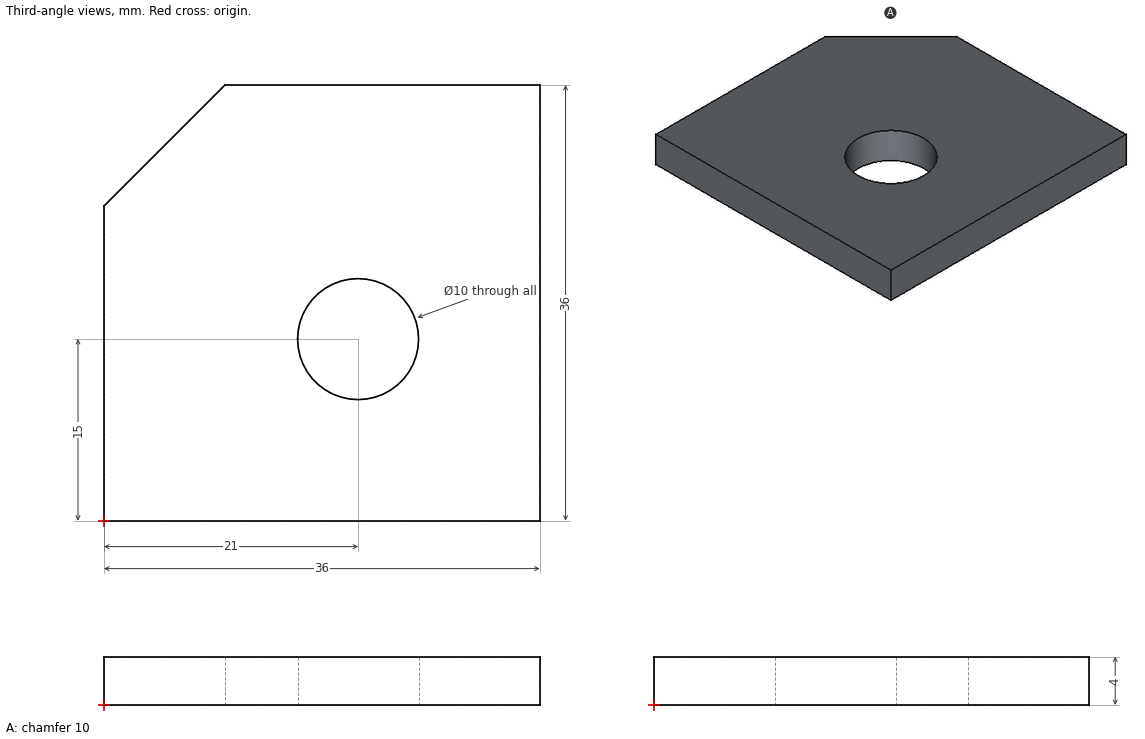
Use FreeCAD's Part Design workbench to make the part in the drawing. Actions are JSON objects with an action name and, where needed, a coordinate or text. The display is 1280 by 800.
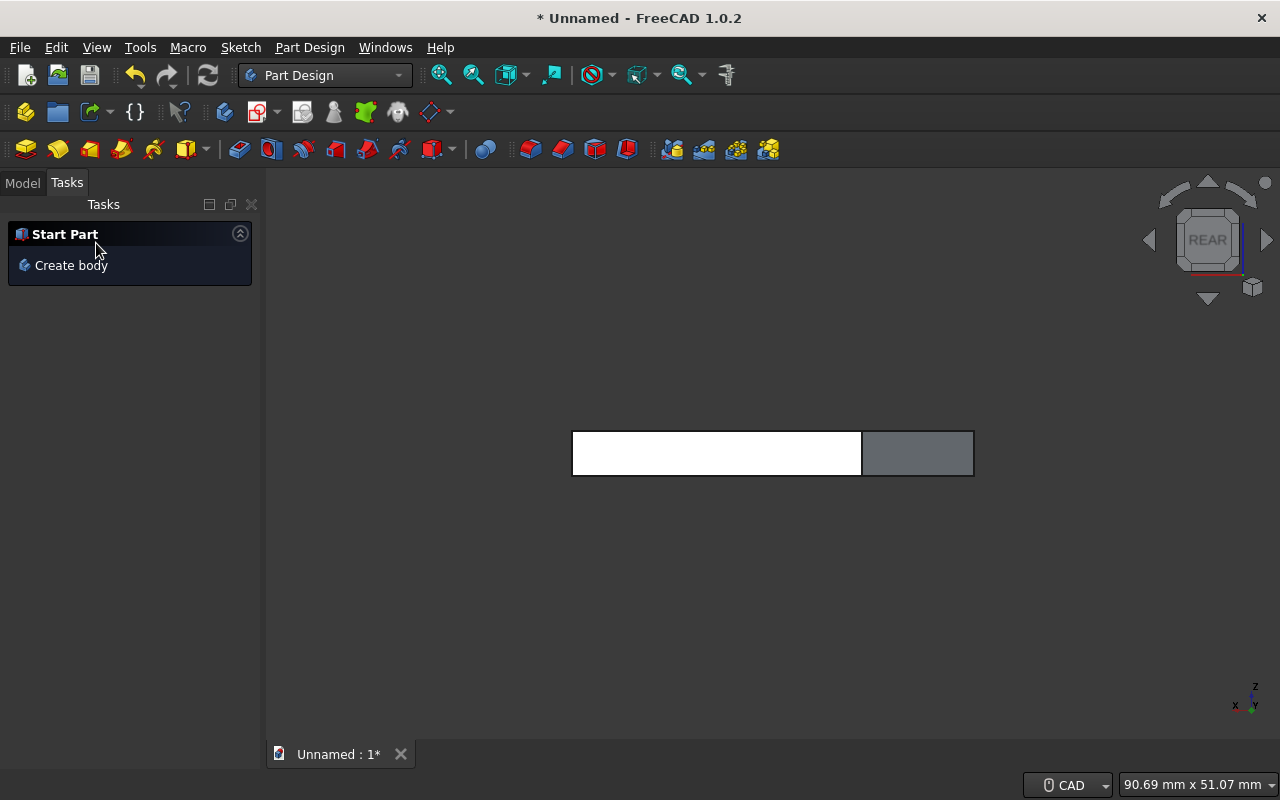
{"action": "key", "text": "v f"}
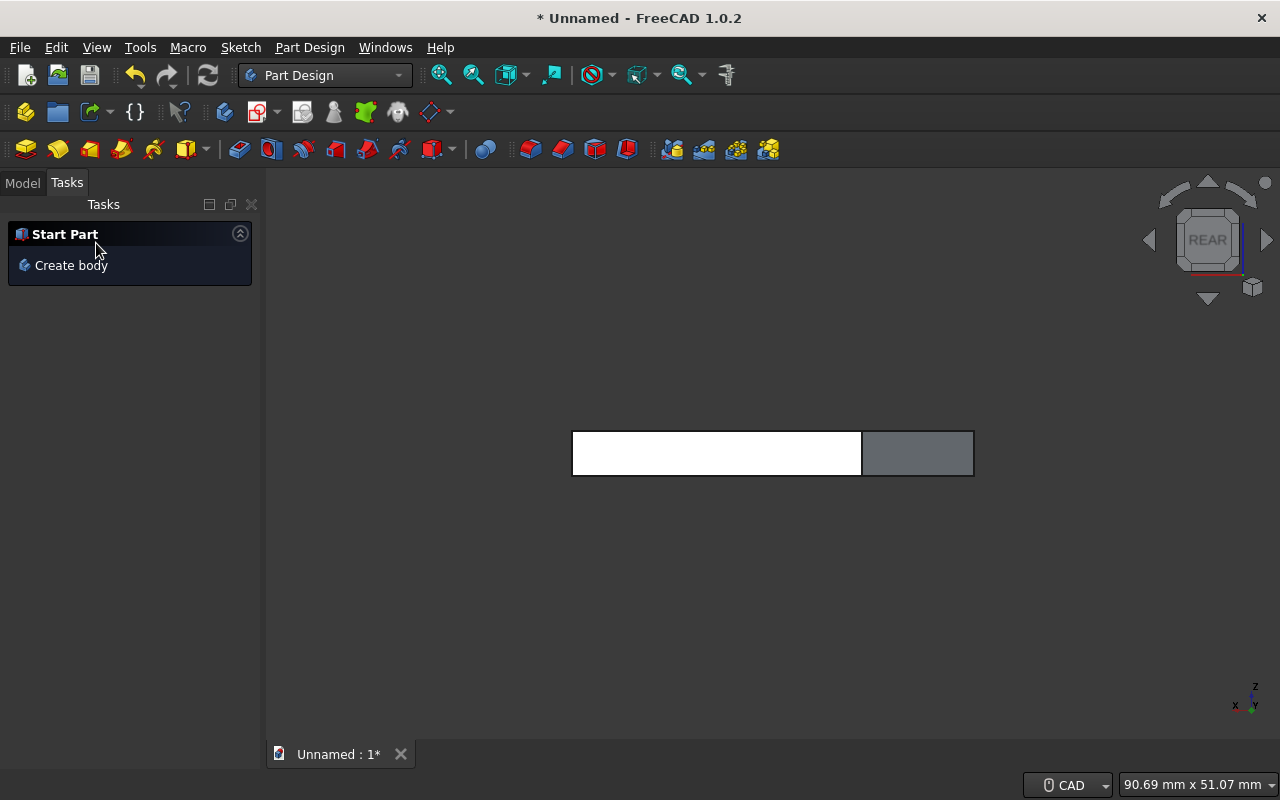
{"action": "key", "text": "0"}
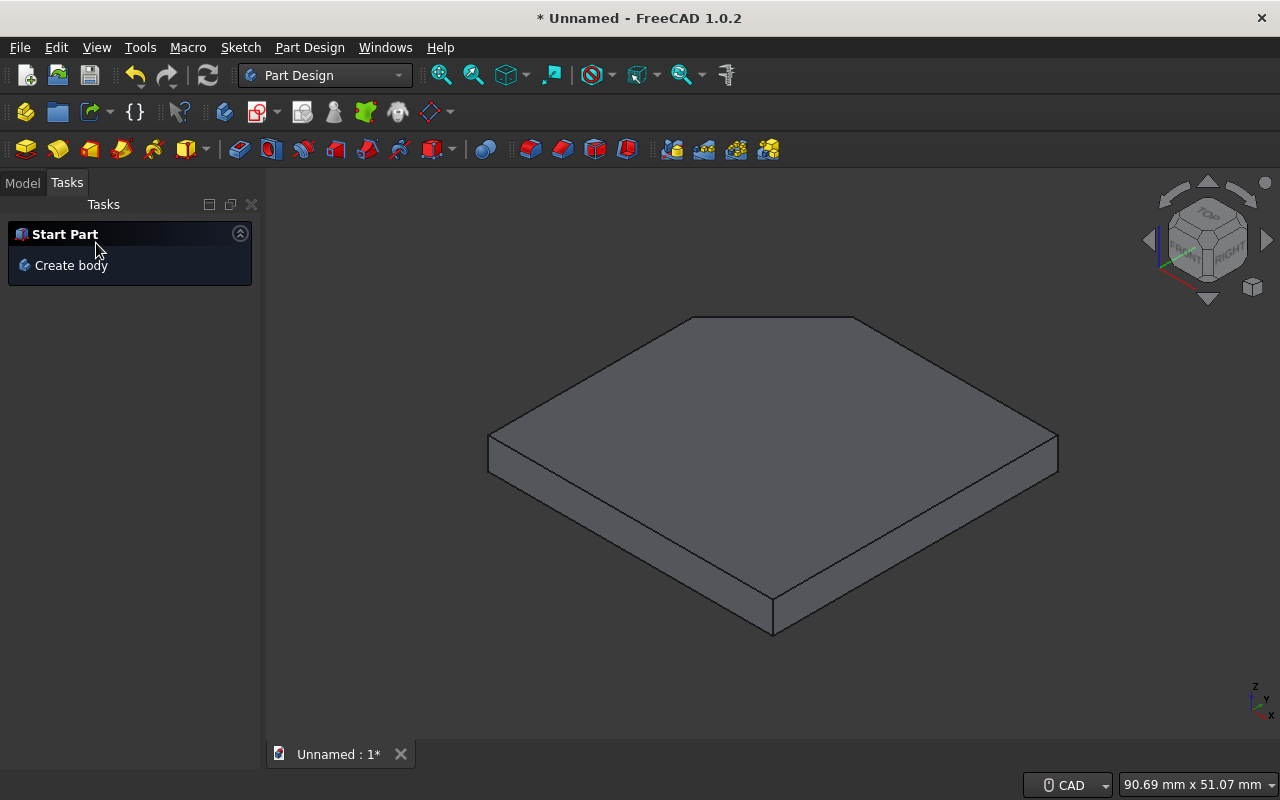
{"action": "left_click", "coordinate": [773, 434]}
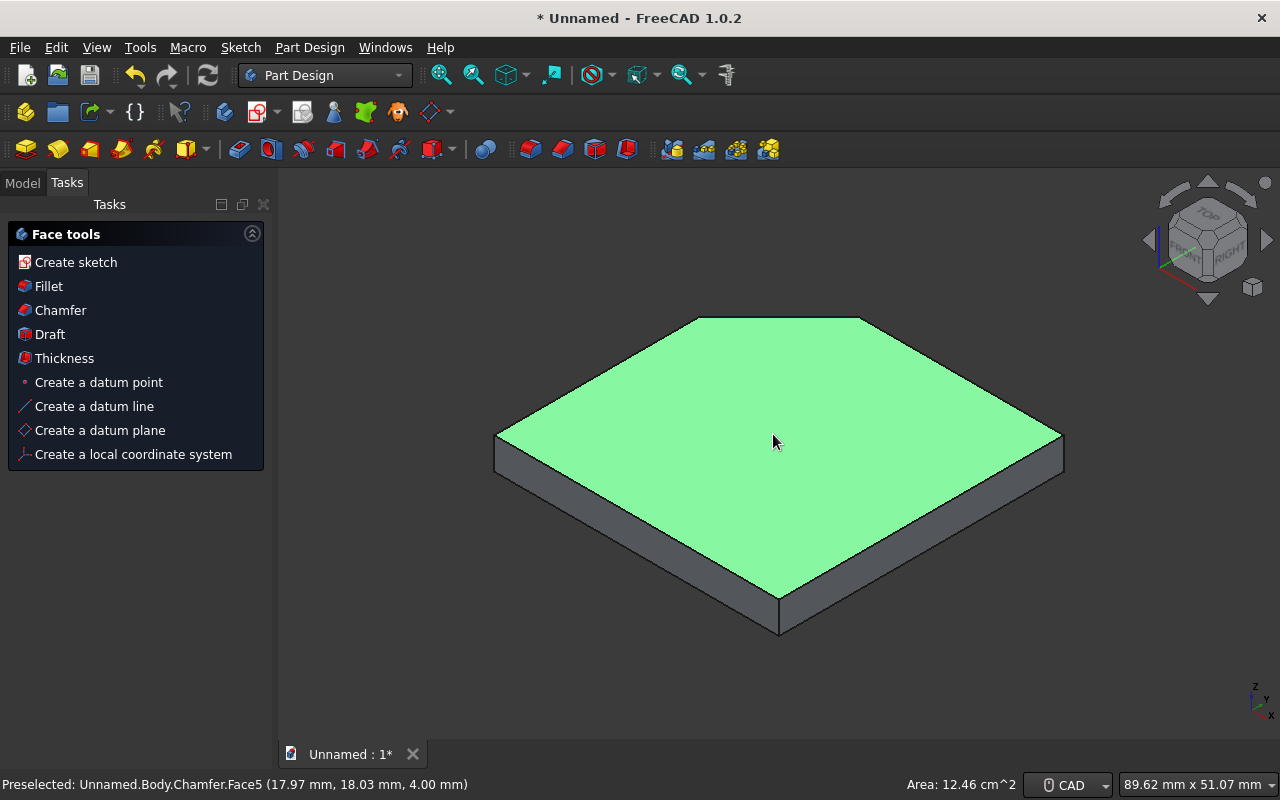
{"action": "left_click", "coordinate": [258, 112]}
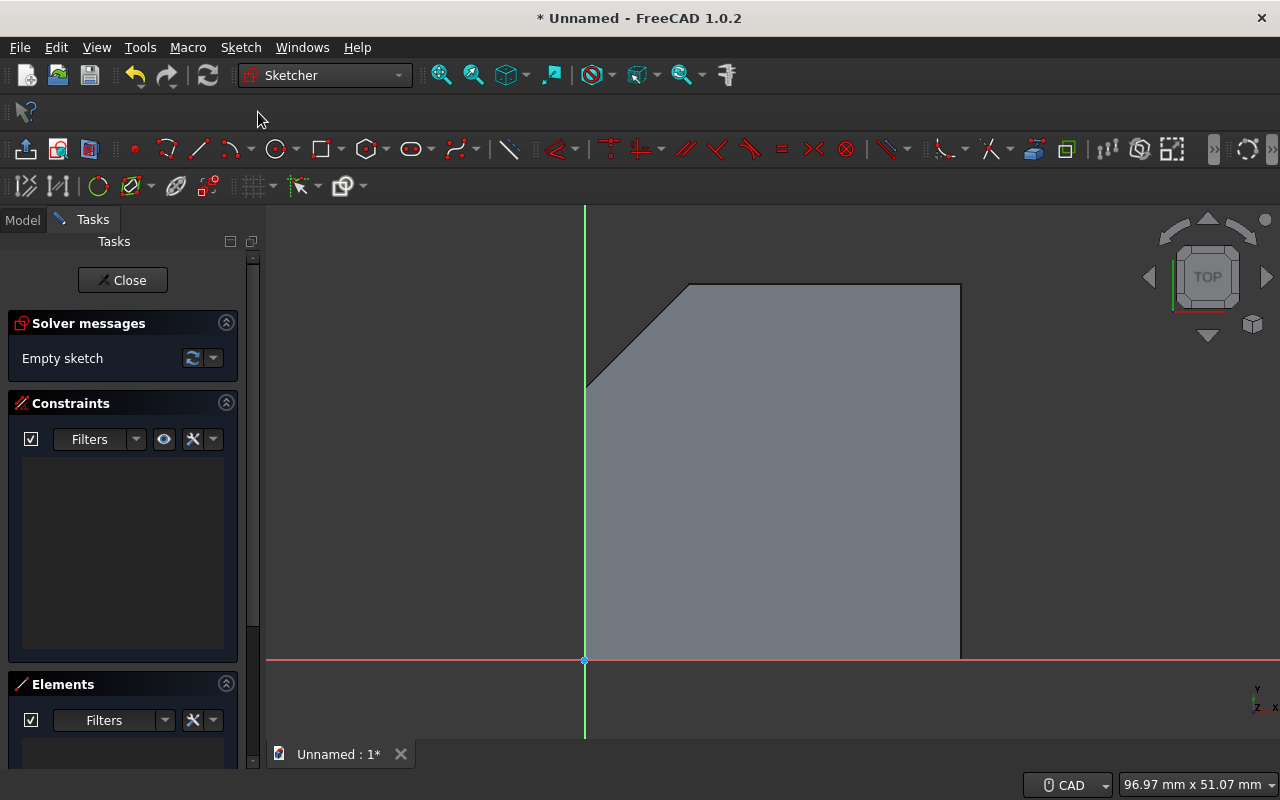
{"action": "scroll", "coordinate": [847, 517], "scroll_direction": "up", "scroll_amount": 6}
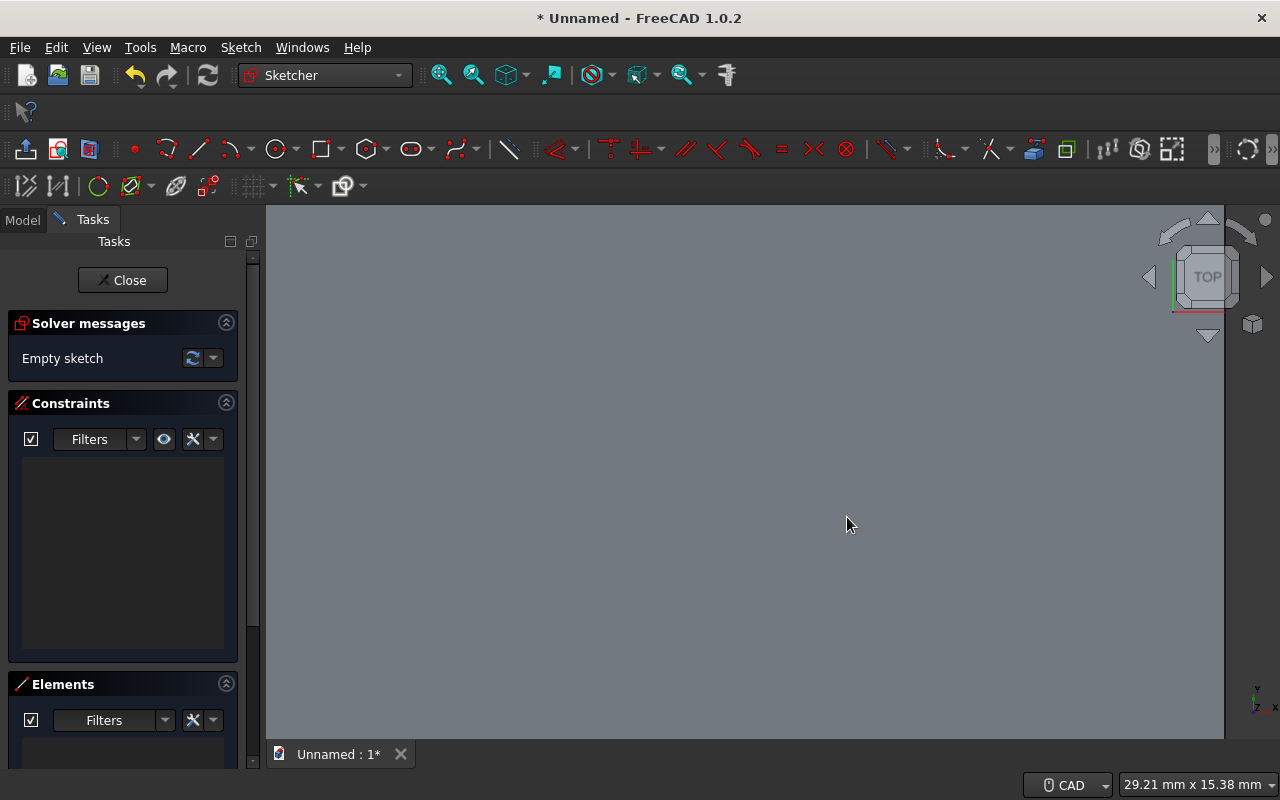
{"action": "key", "text": "g c"}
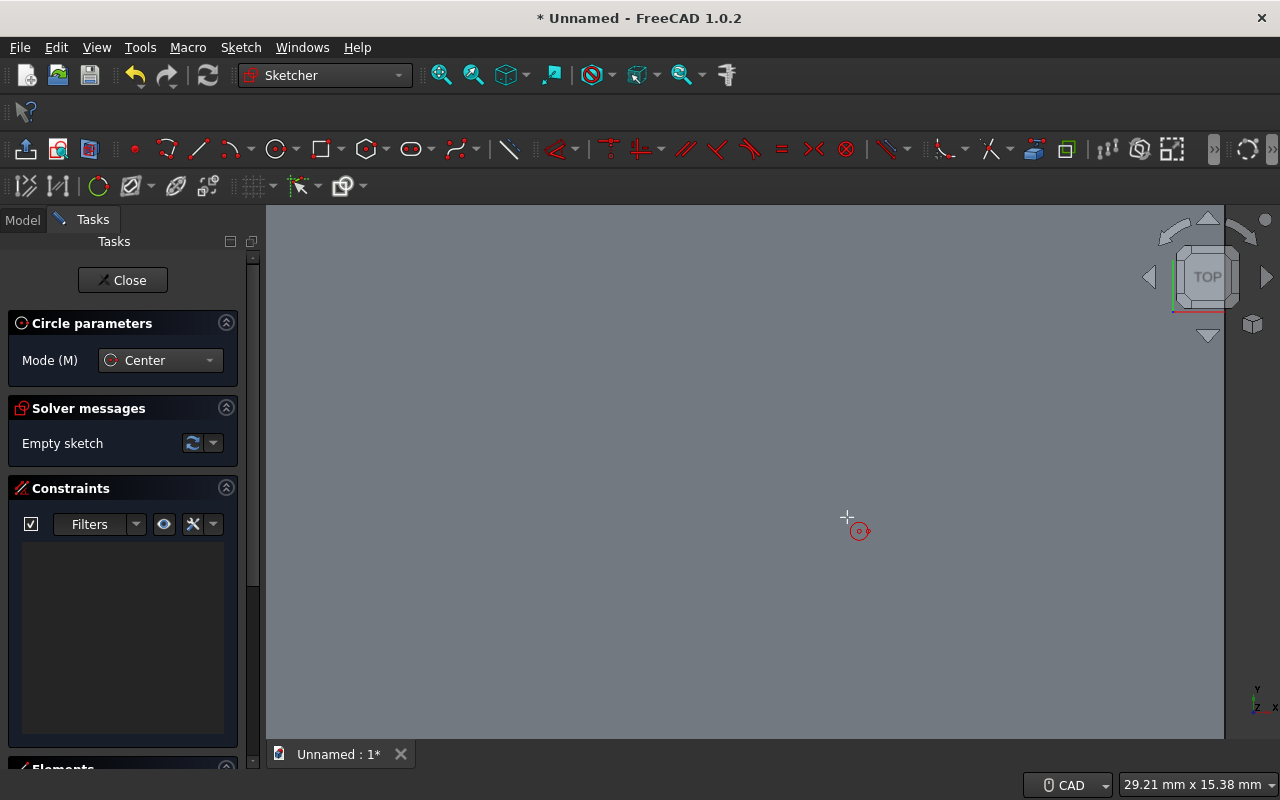
{"action": "left_click", "coordinate": [704, 470]}
{"action": "left_click", "coordinate": [827, 348]}
{"action": "key", "text": "Escape"}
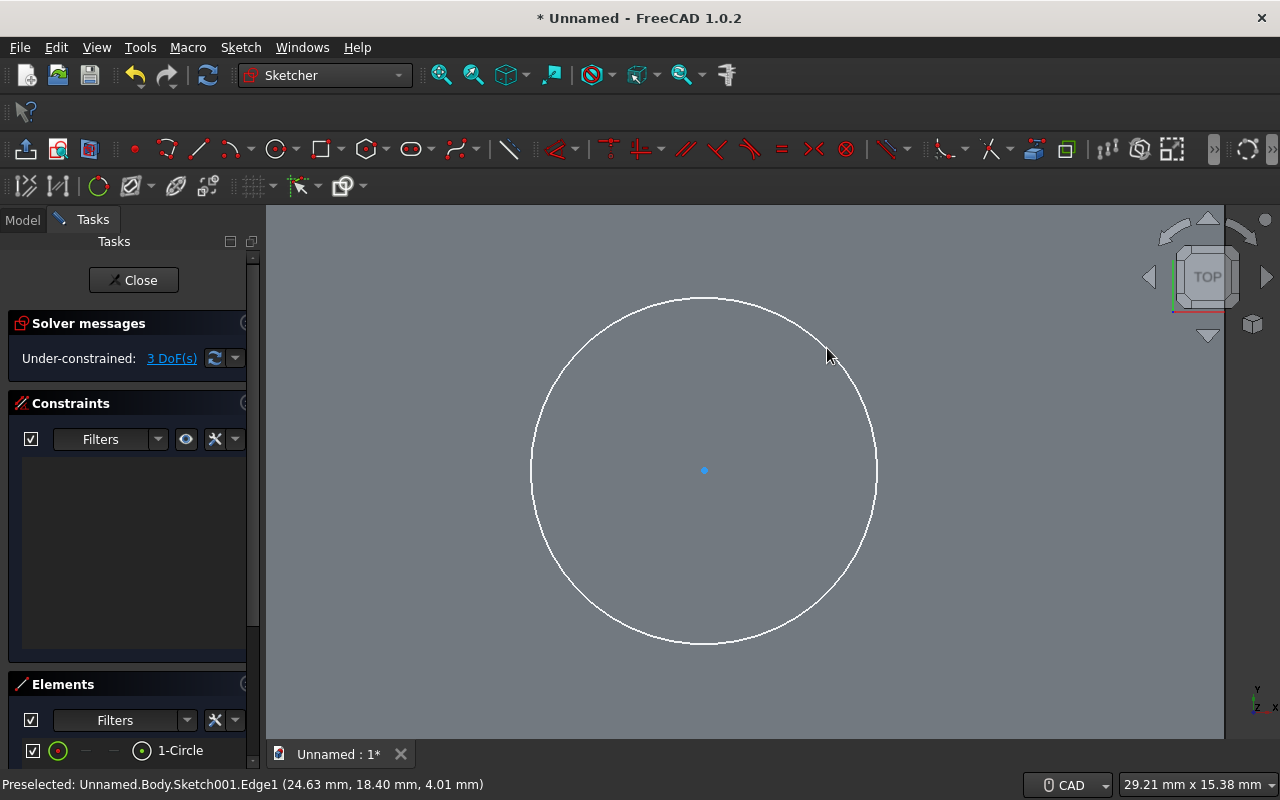
{"action": "left_click", "coordinate": [556, 150]}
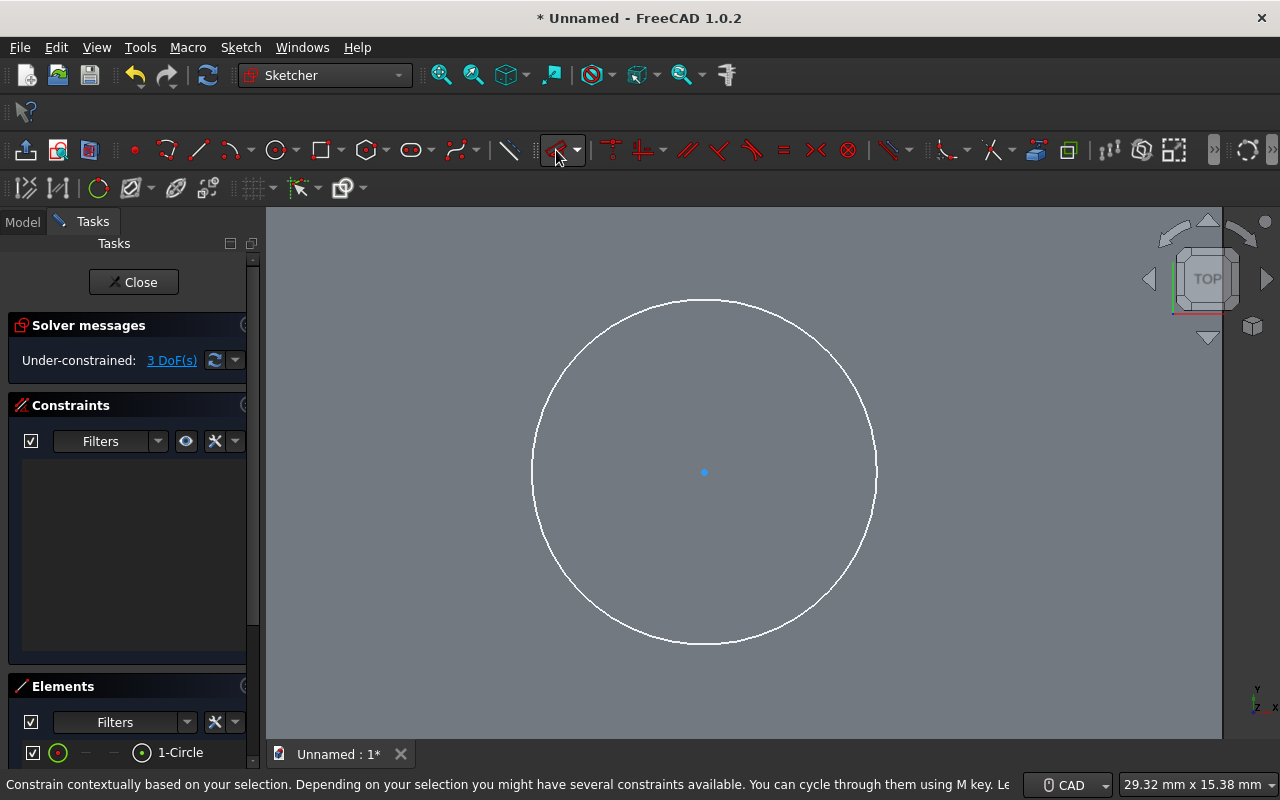
{"action": "left_click", "coordinate": [826, 350]}
{"action": "left_click", "coordinate": [849, 327]}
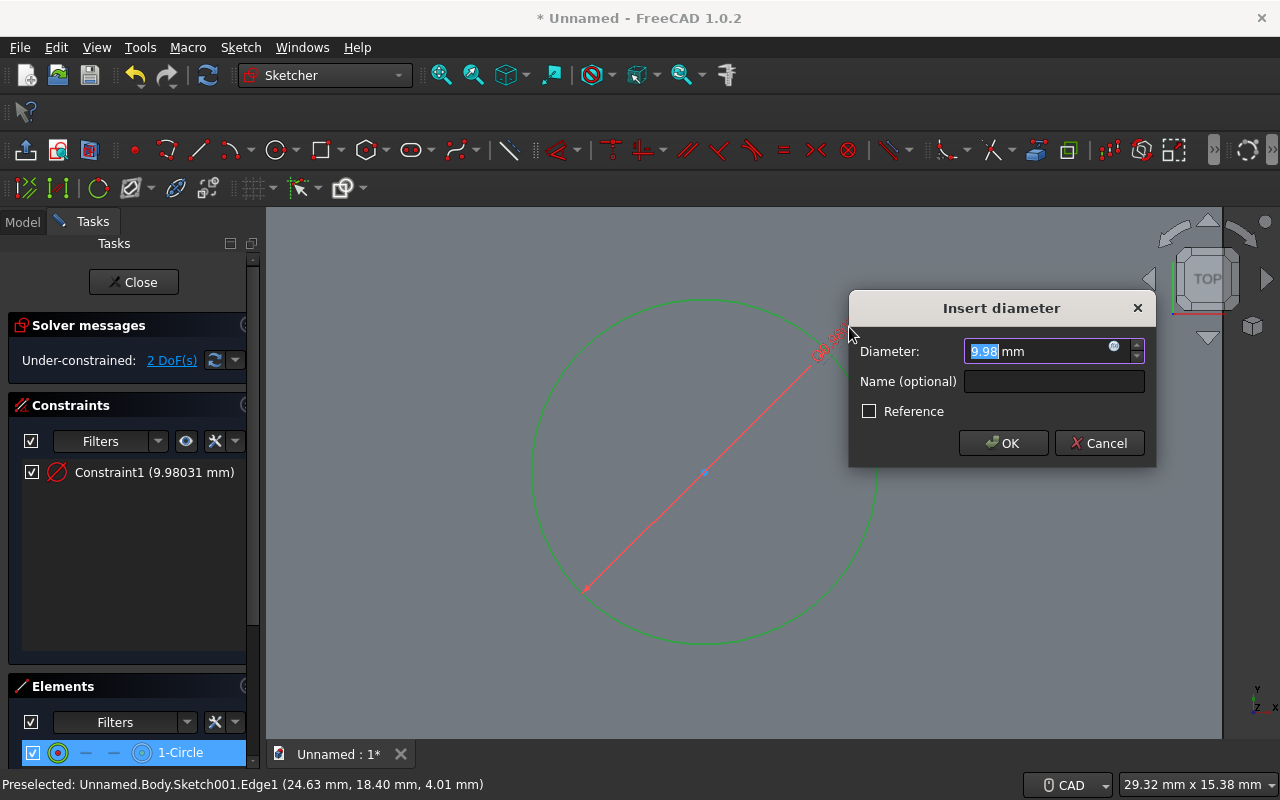
{"action": "type", "text": "10"}
{"action": "key", "text": "Return"}